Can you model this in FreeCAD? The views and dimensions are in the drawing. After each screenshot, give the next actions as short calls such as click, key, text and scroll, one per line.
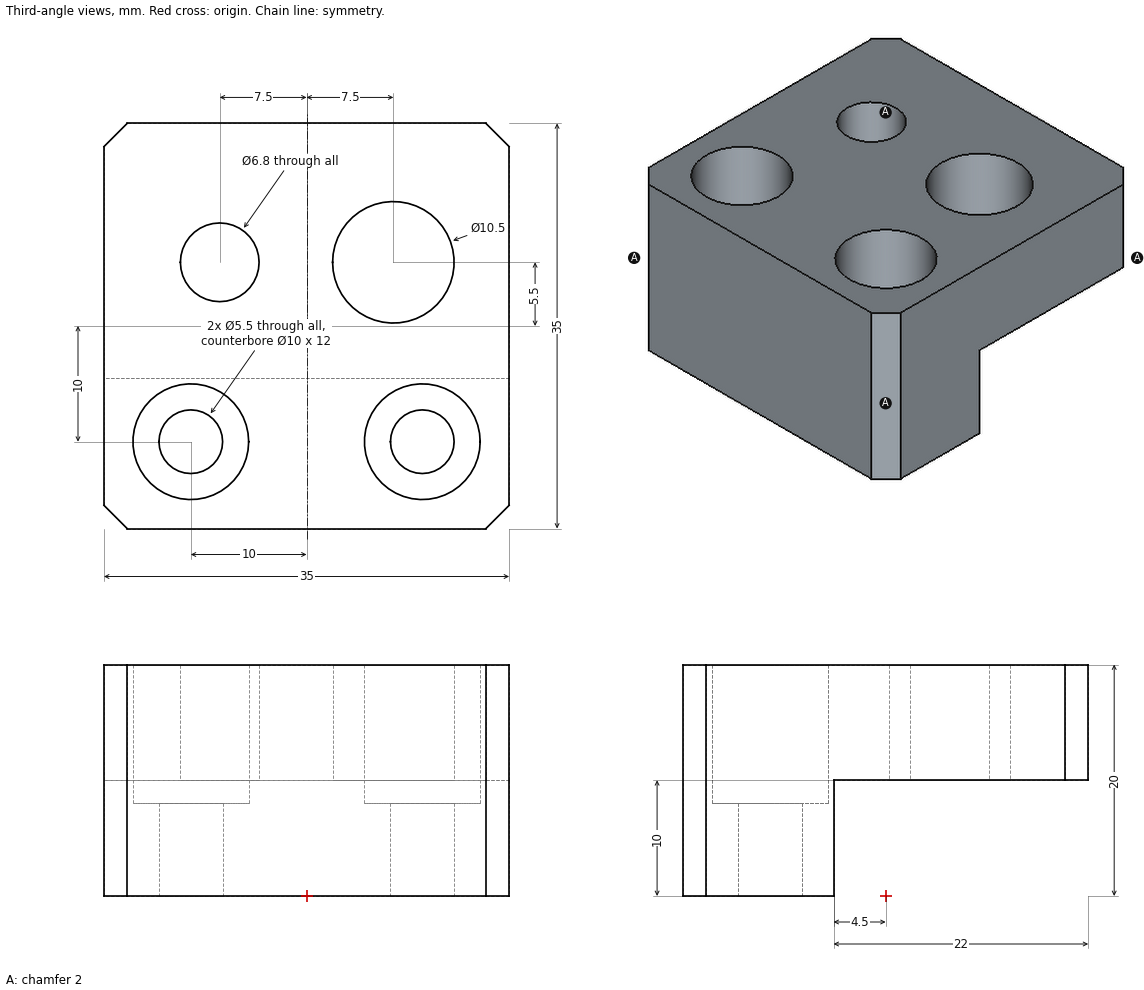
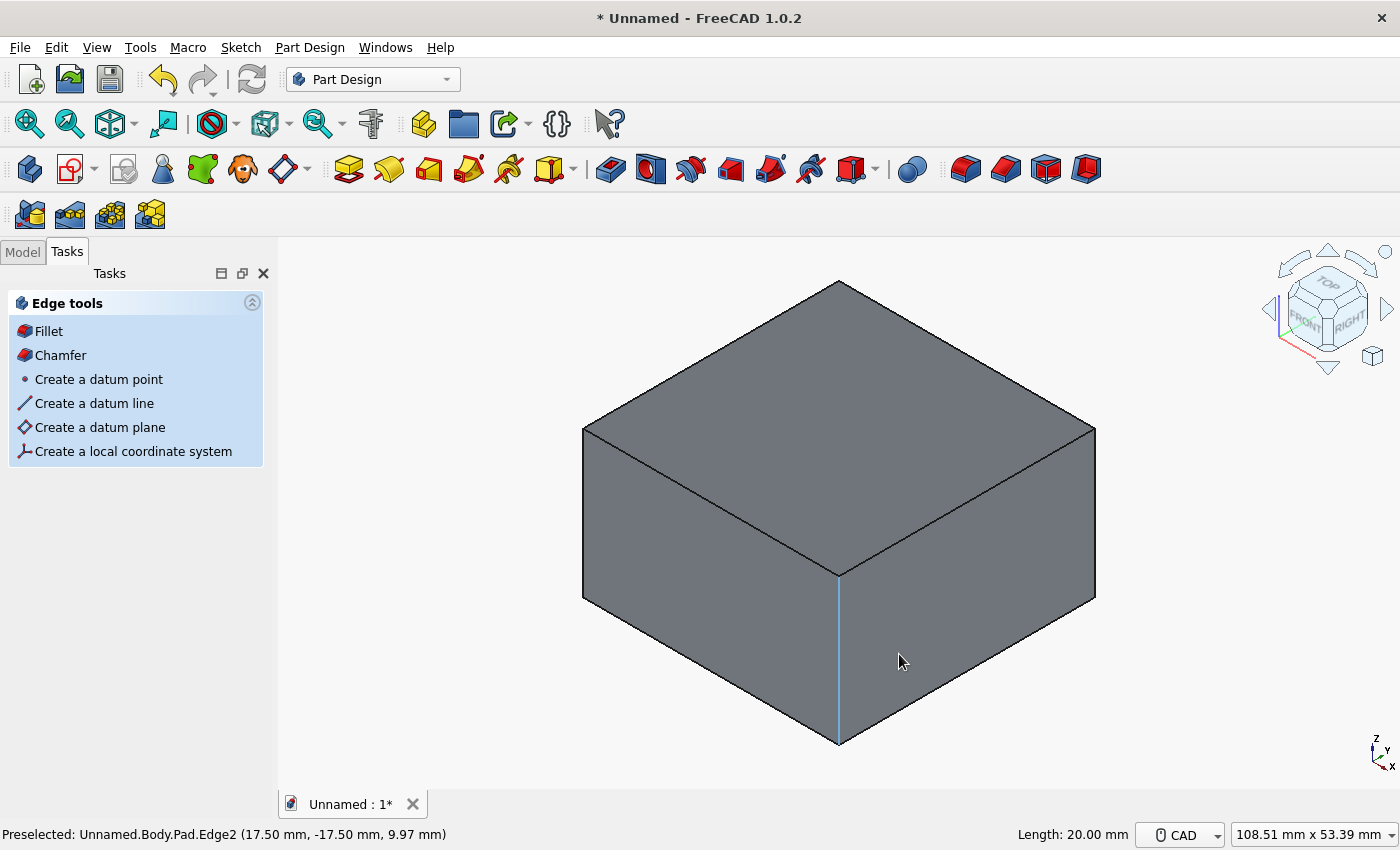
key(2)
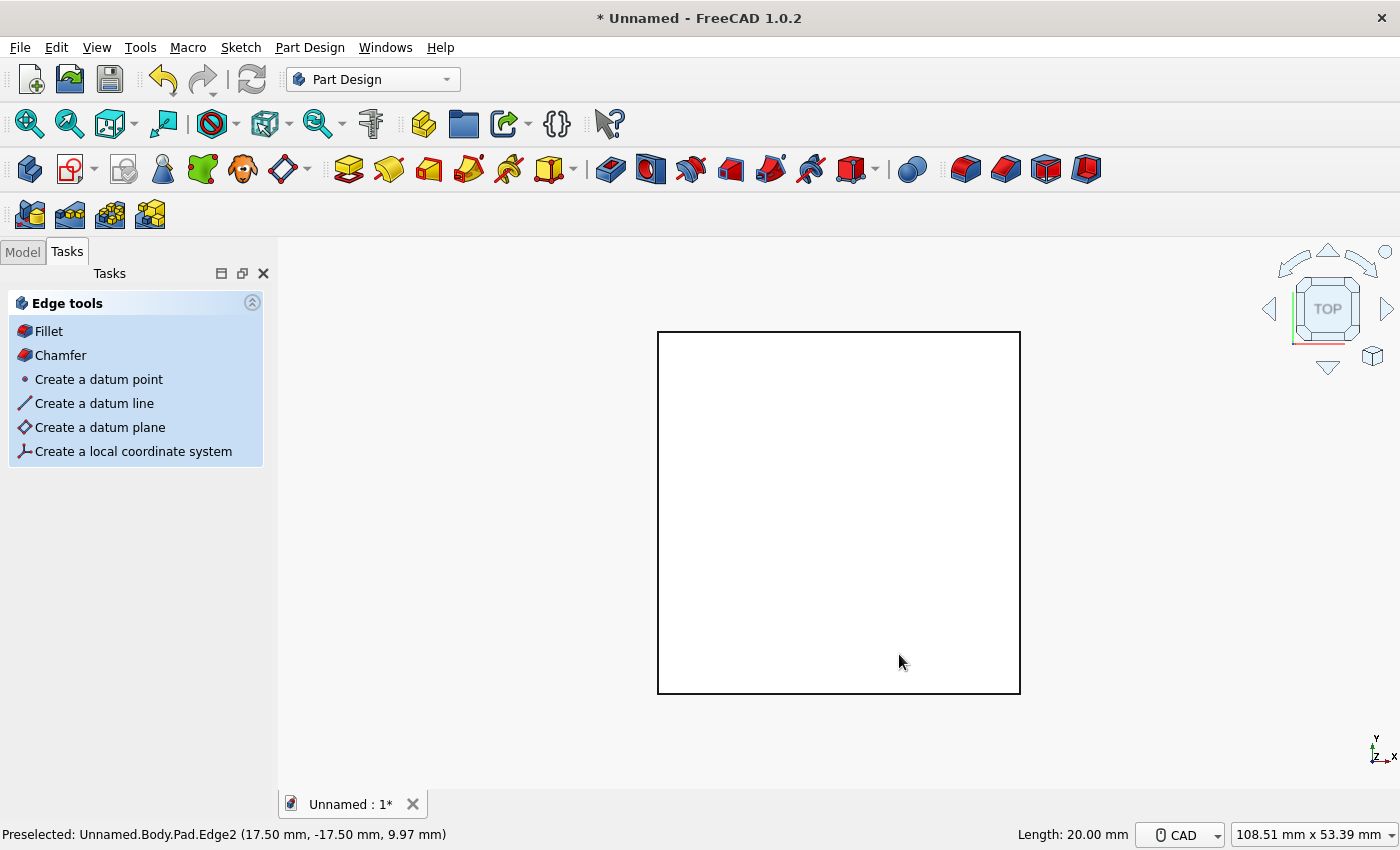
key(1)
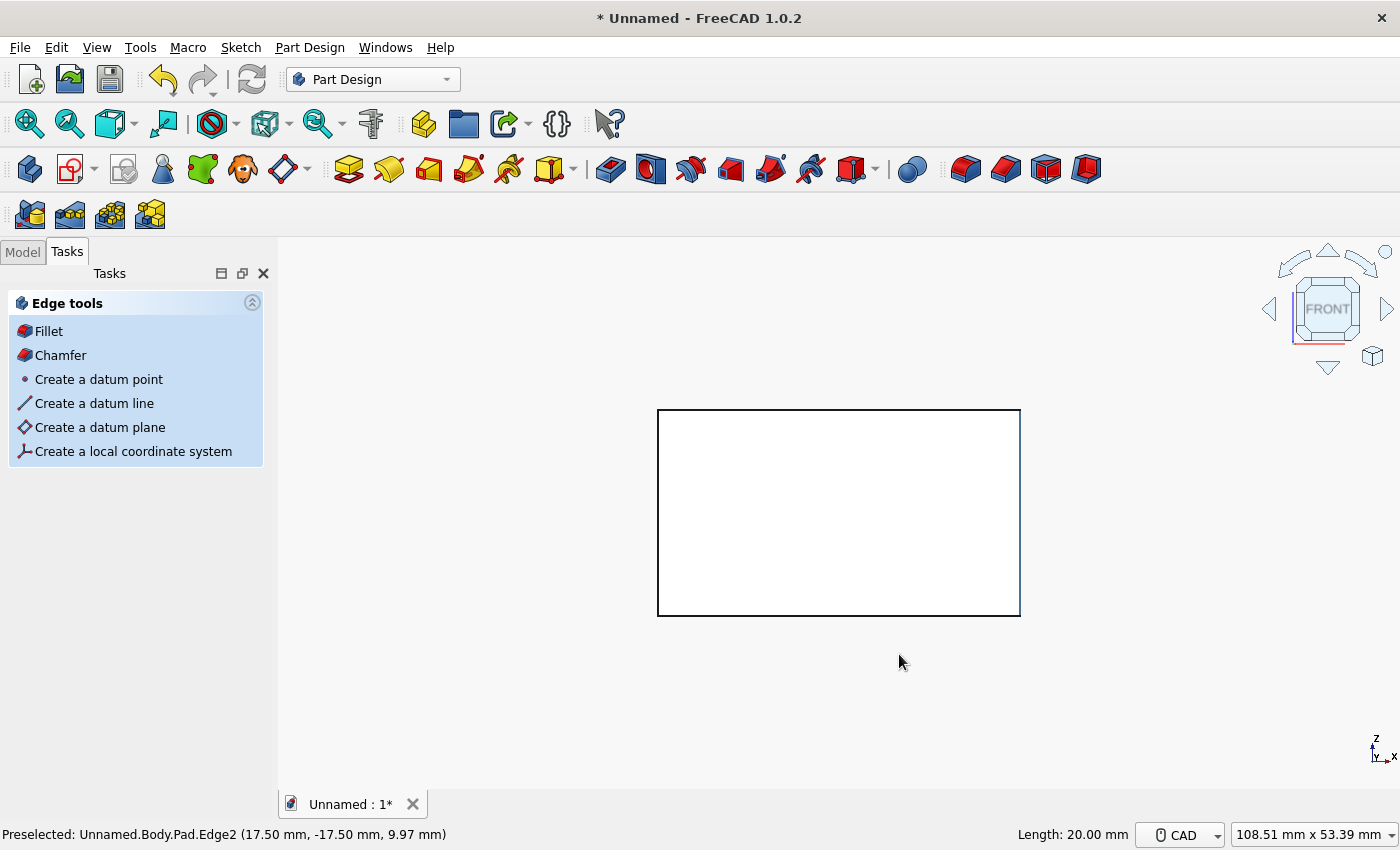
key(v)
key(f)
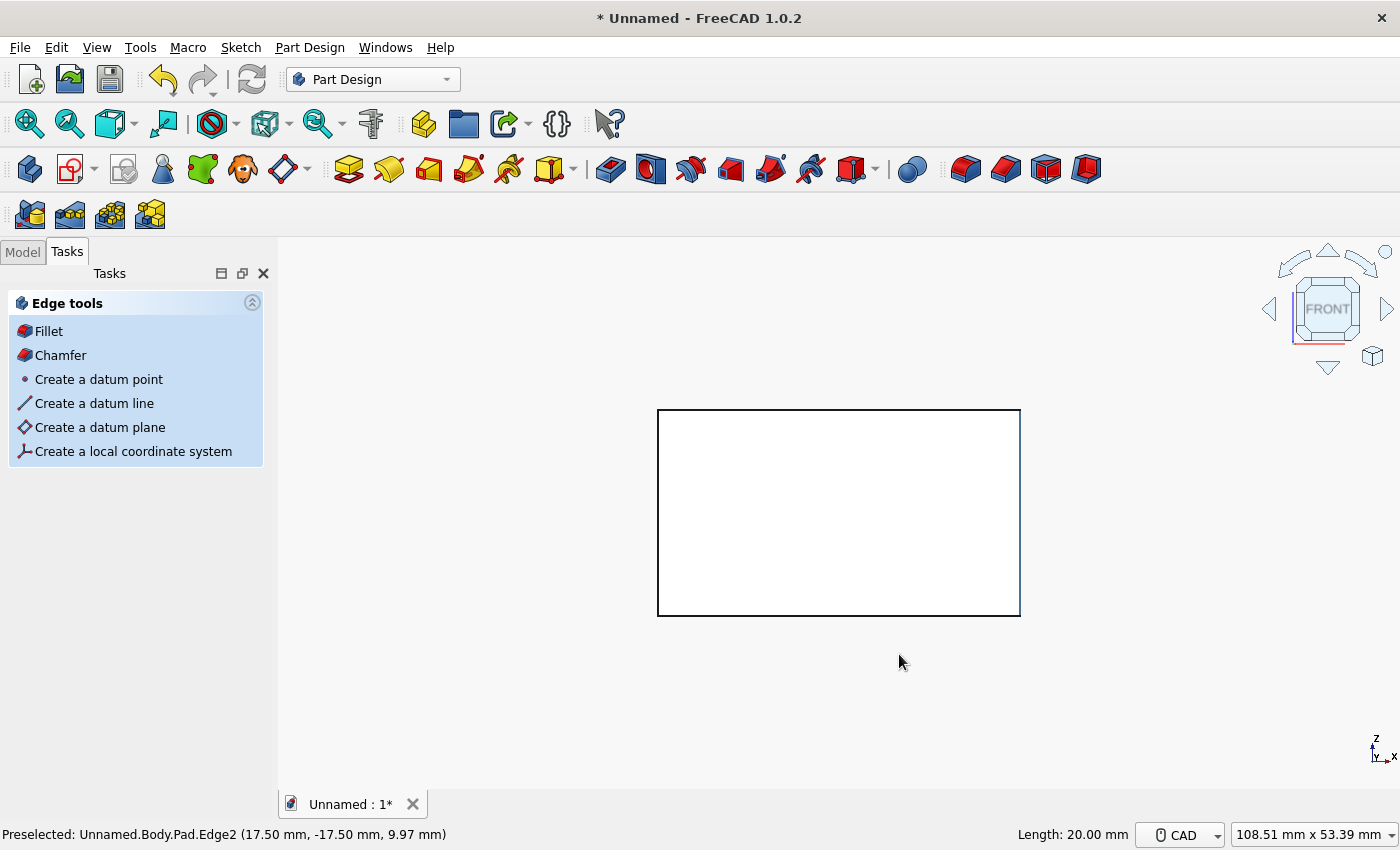
click(658, 512, ctrl)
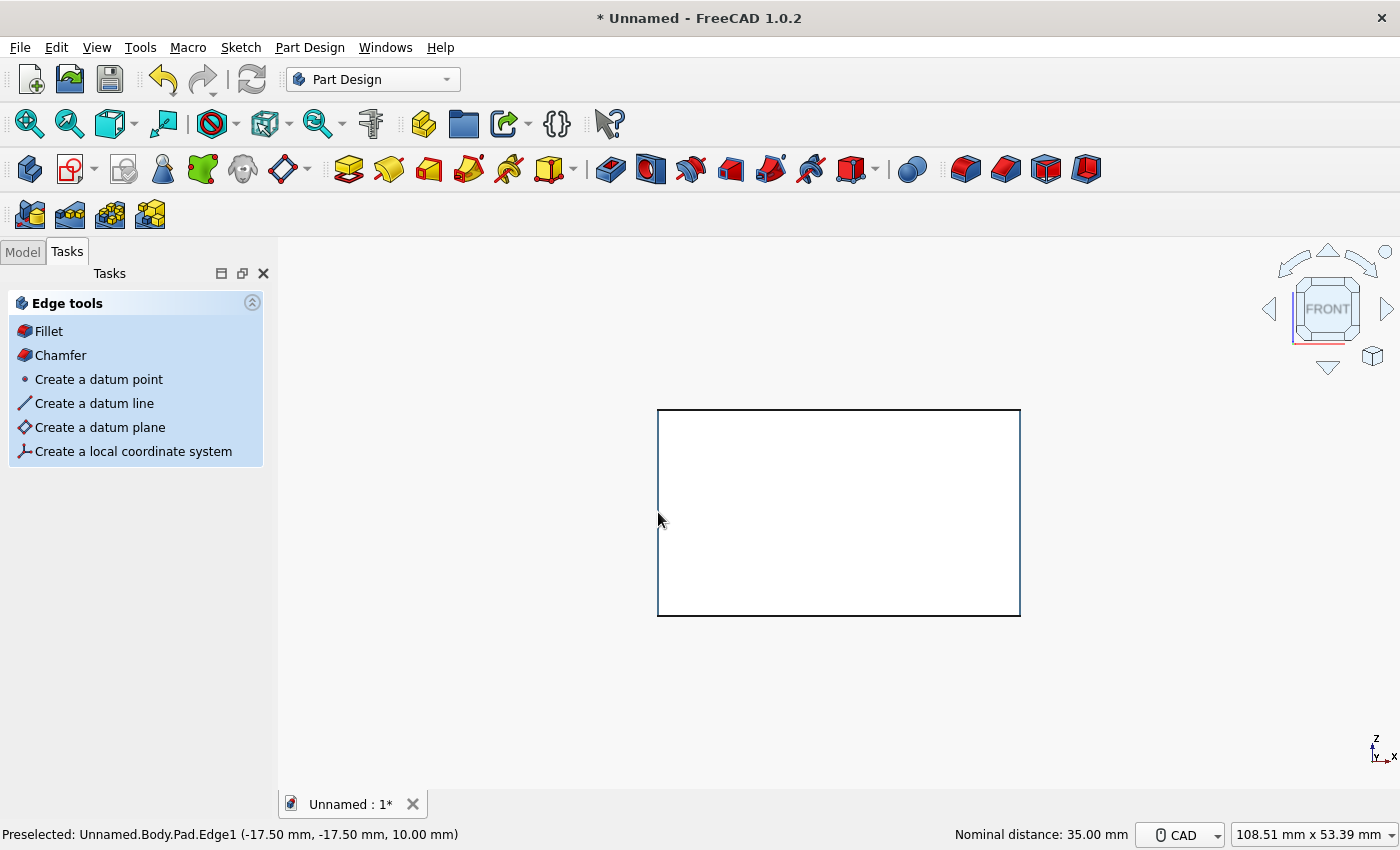
key(3)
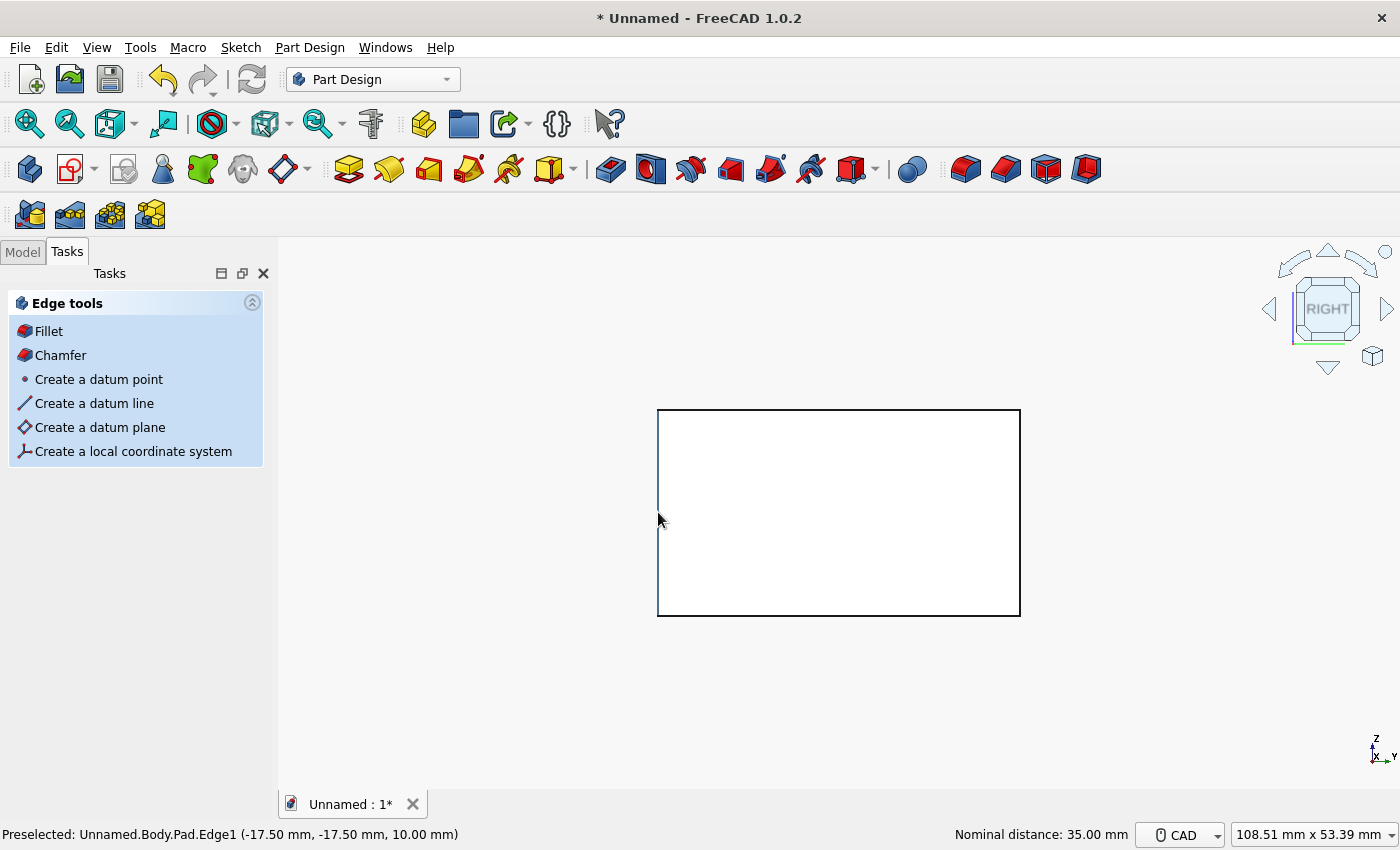
key(v)
key(f)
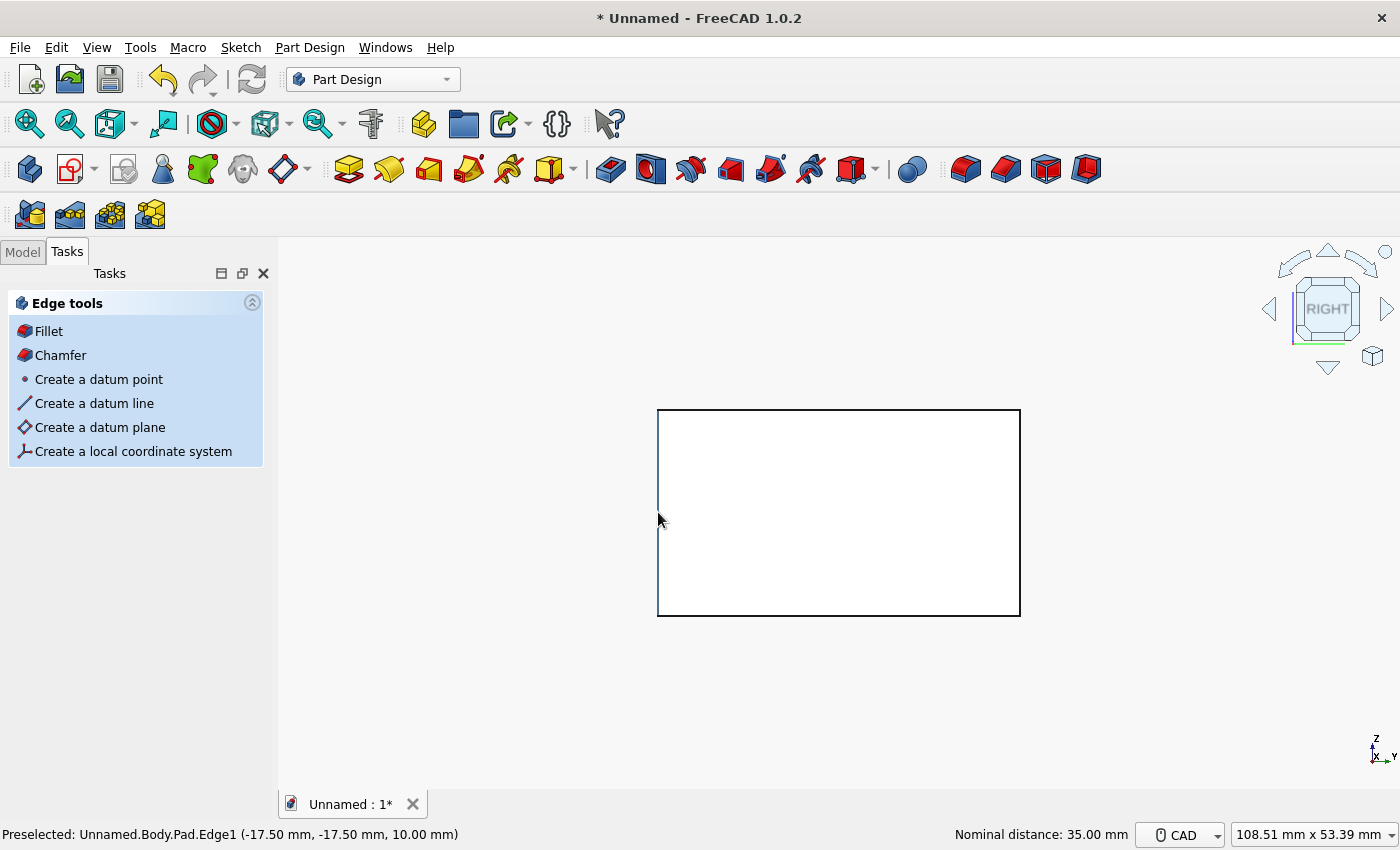
click(1020, 512, ctrl)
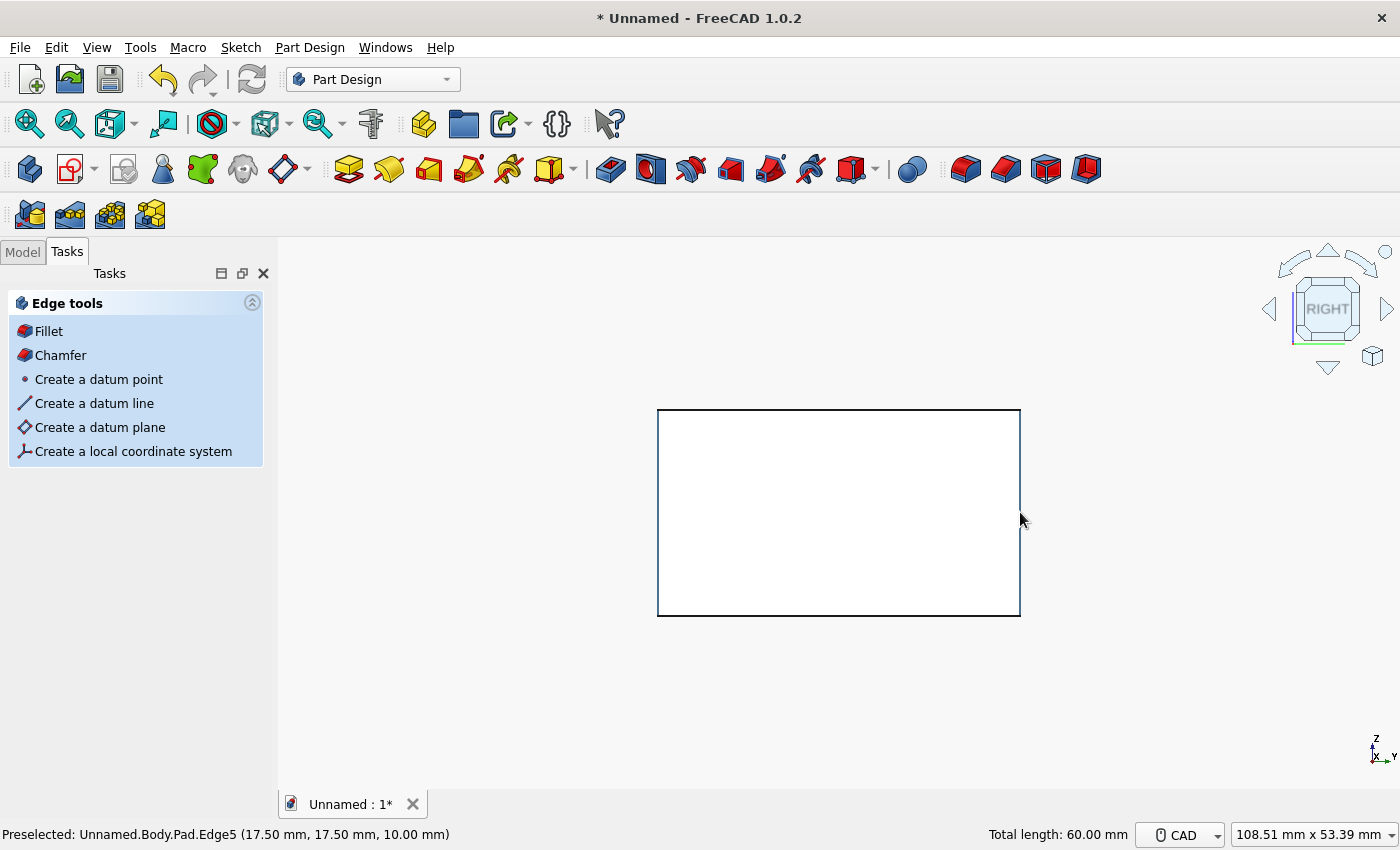
key(5)